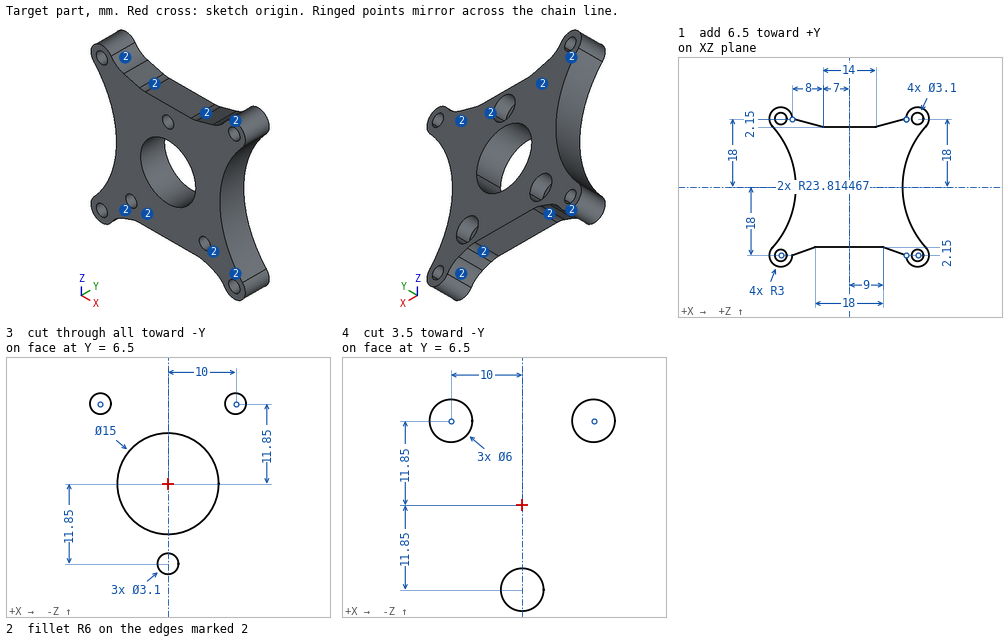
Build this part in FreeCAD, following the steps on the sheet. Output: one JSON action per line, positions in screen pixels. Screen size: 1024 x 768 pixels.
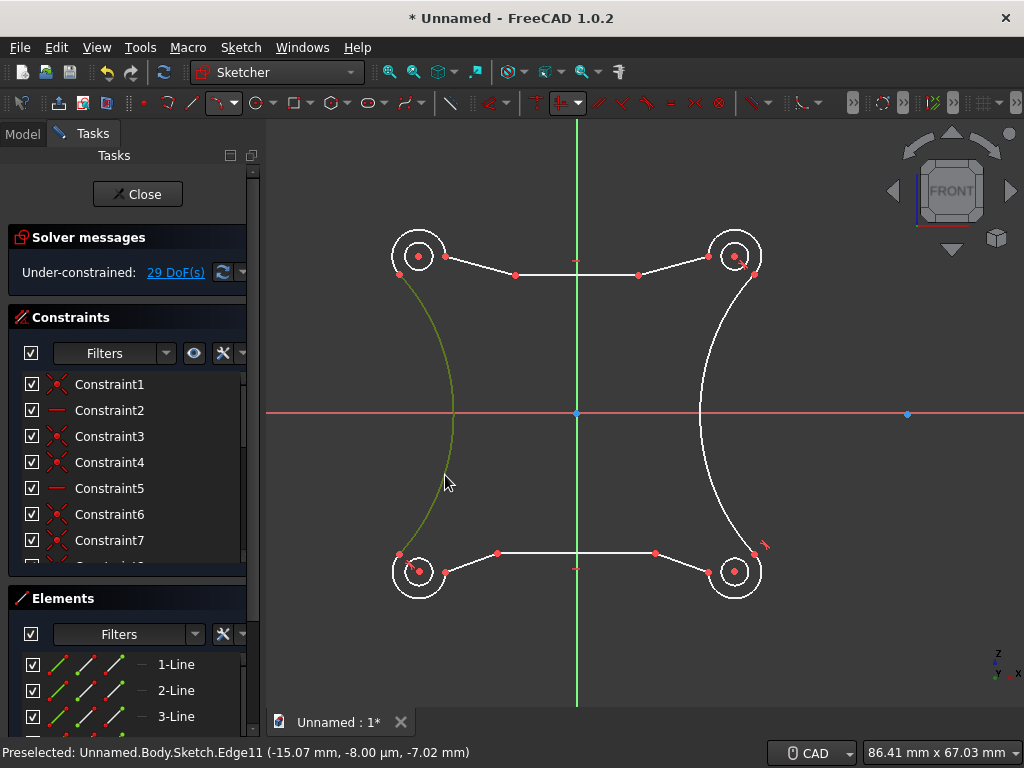
{"action": "left_click", "coordinate": [429, 232]}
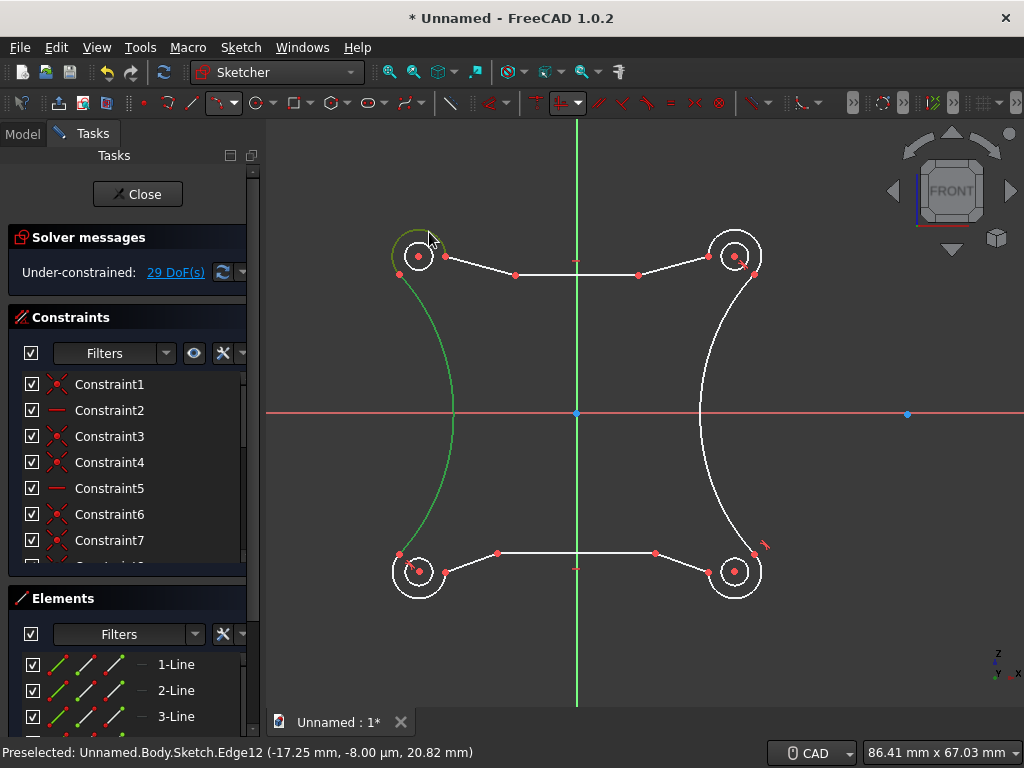
{"action": "left_click", "coordinate": [648, 104]}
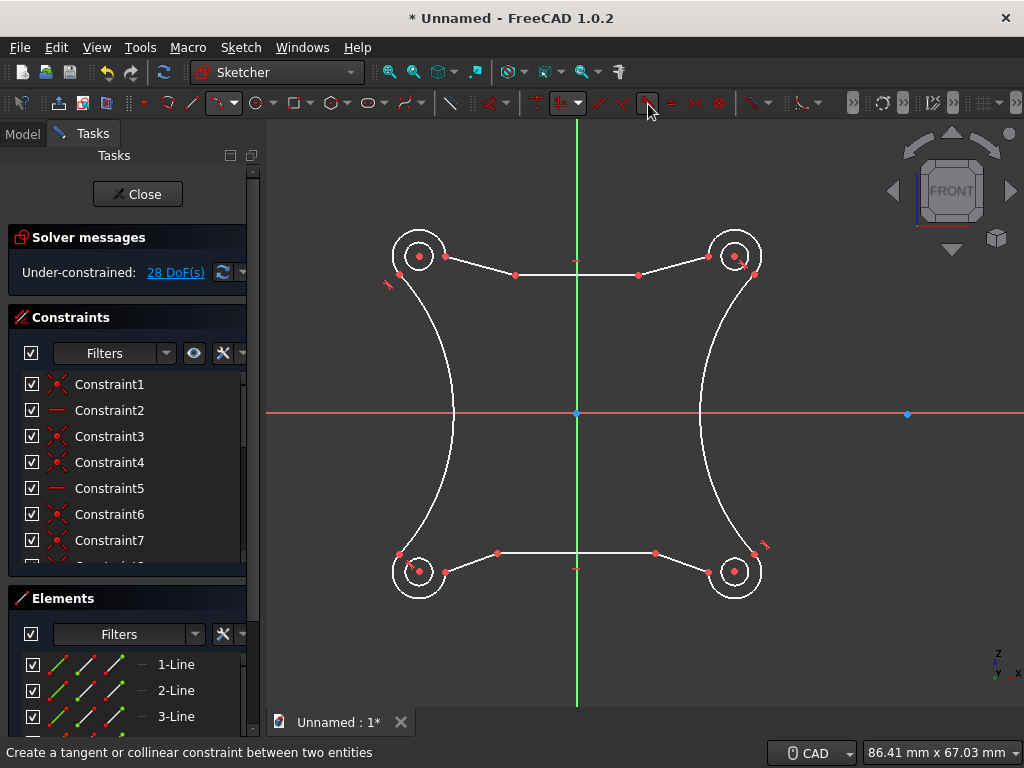
{"action": "left_click", "coordinate": [759, 245]}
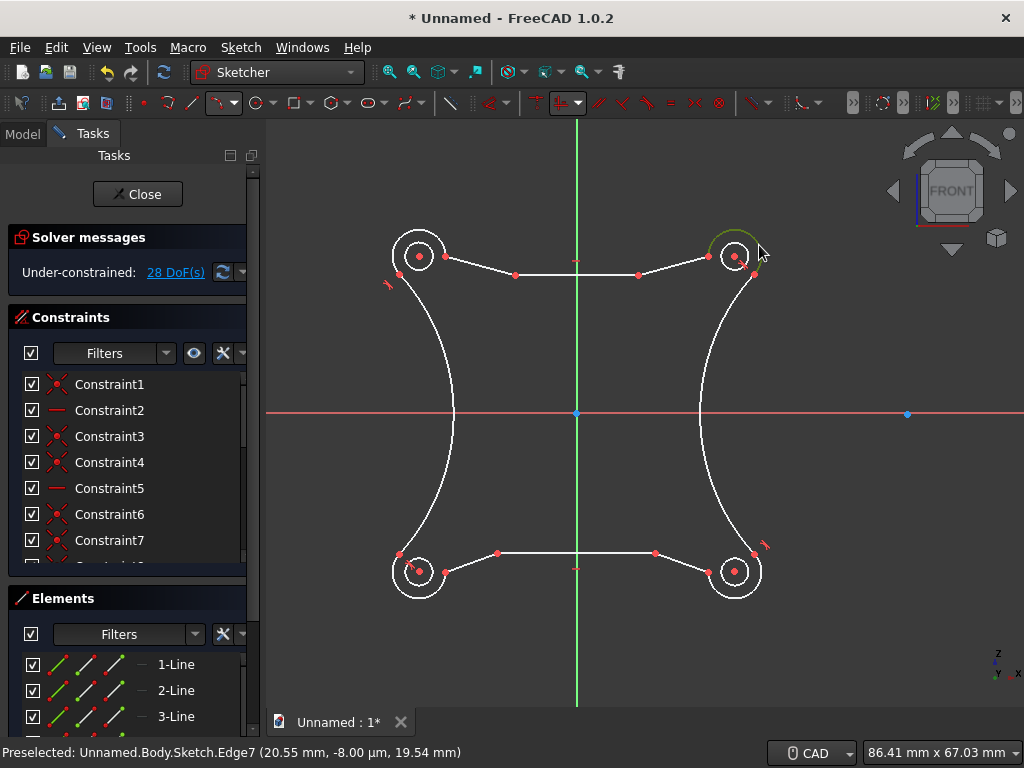
{"action": "left_click", "coordinate": [725, 596]}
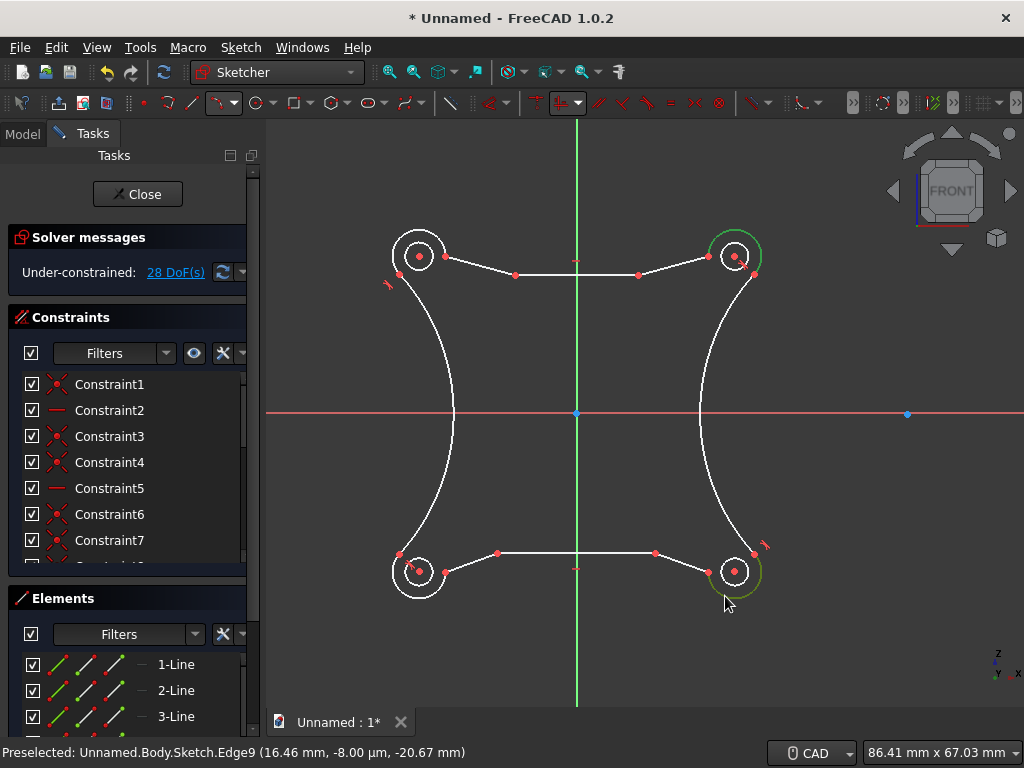
{"action": "left_click", "coordinate": [395, 583]}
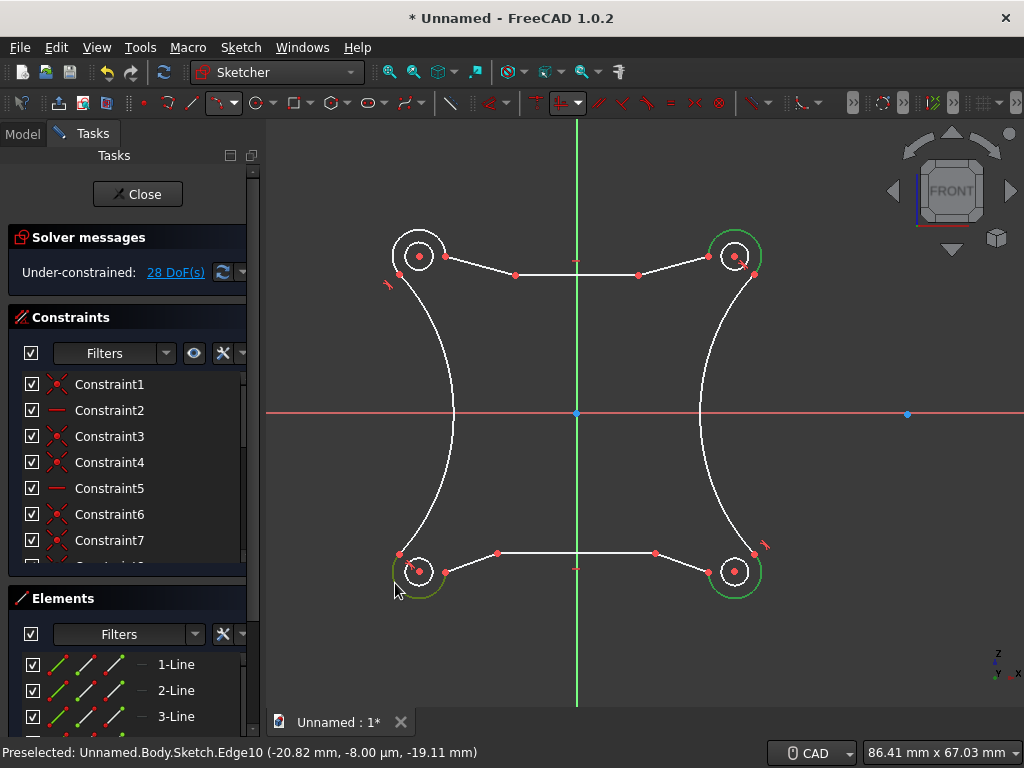
{"action": "left_click", "coordinate": [430, 232]}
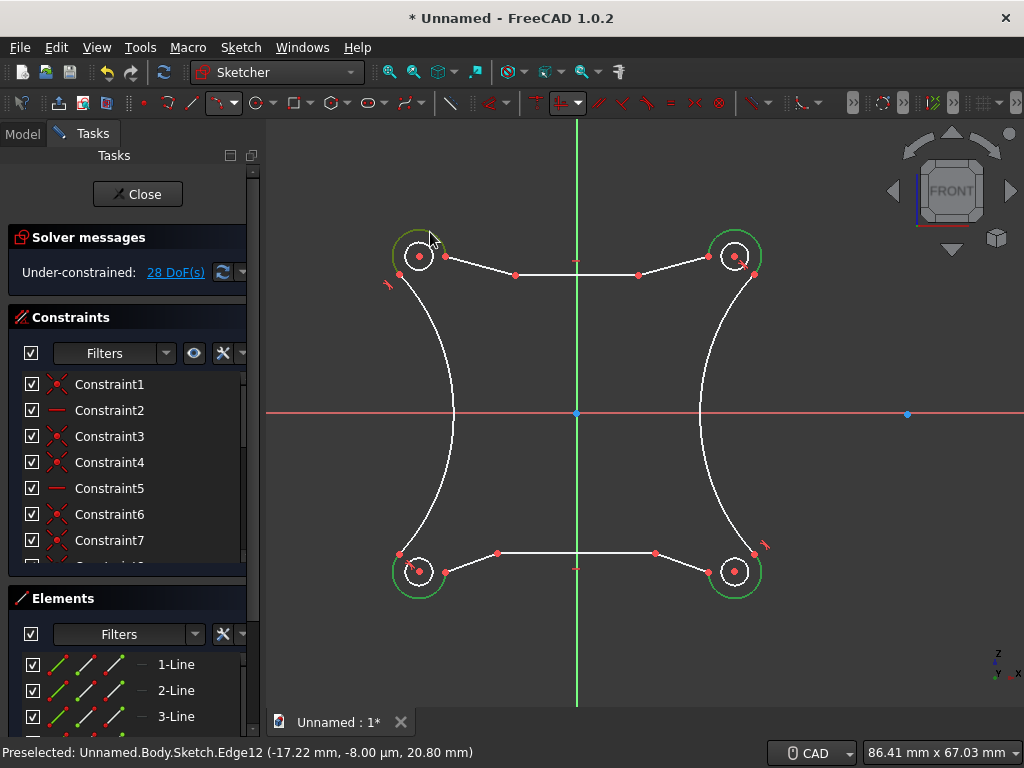
{"action": "left_click", "coordinate": [672, 104]}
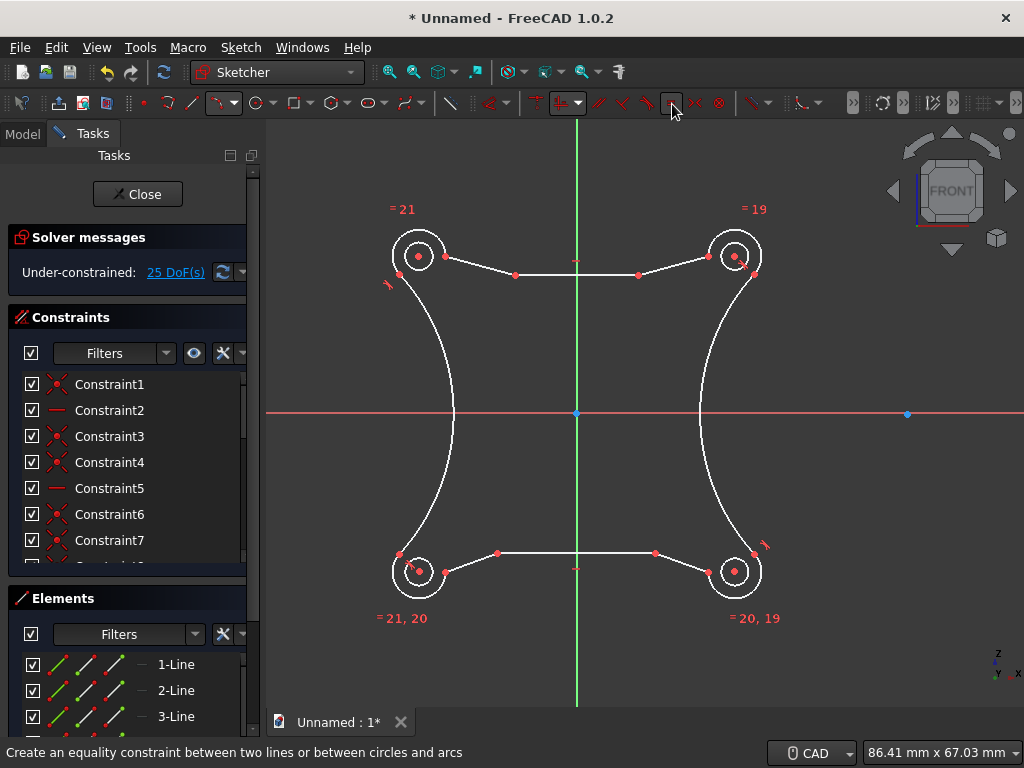
{"action": "left_click", "coordinate": [709, 354]}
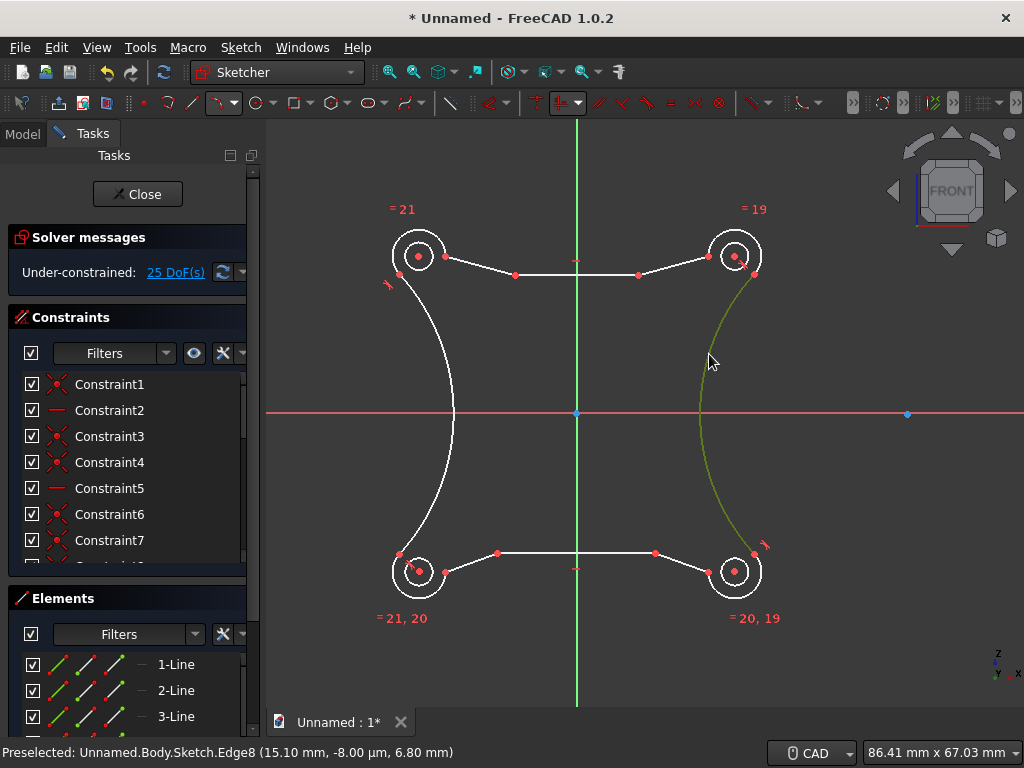
{"action": "left_click", "coordinate": [445, 475]}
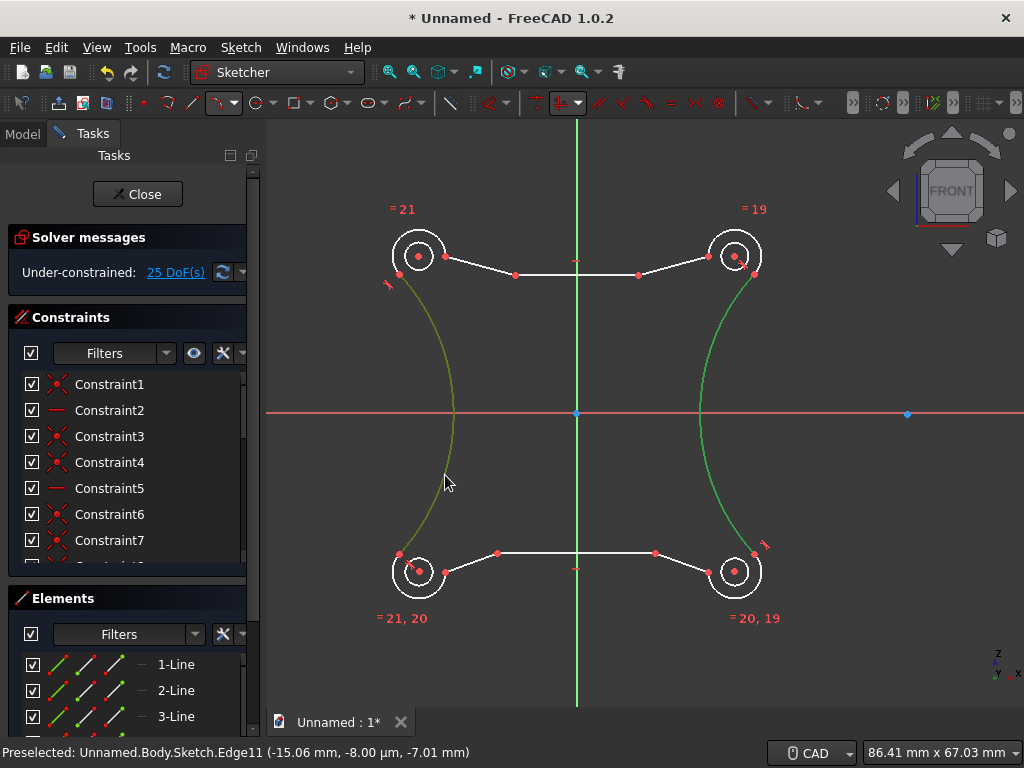
{"action": "left_click", "coordinate": [672, 104]}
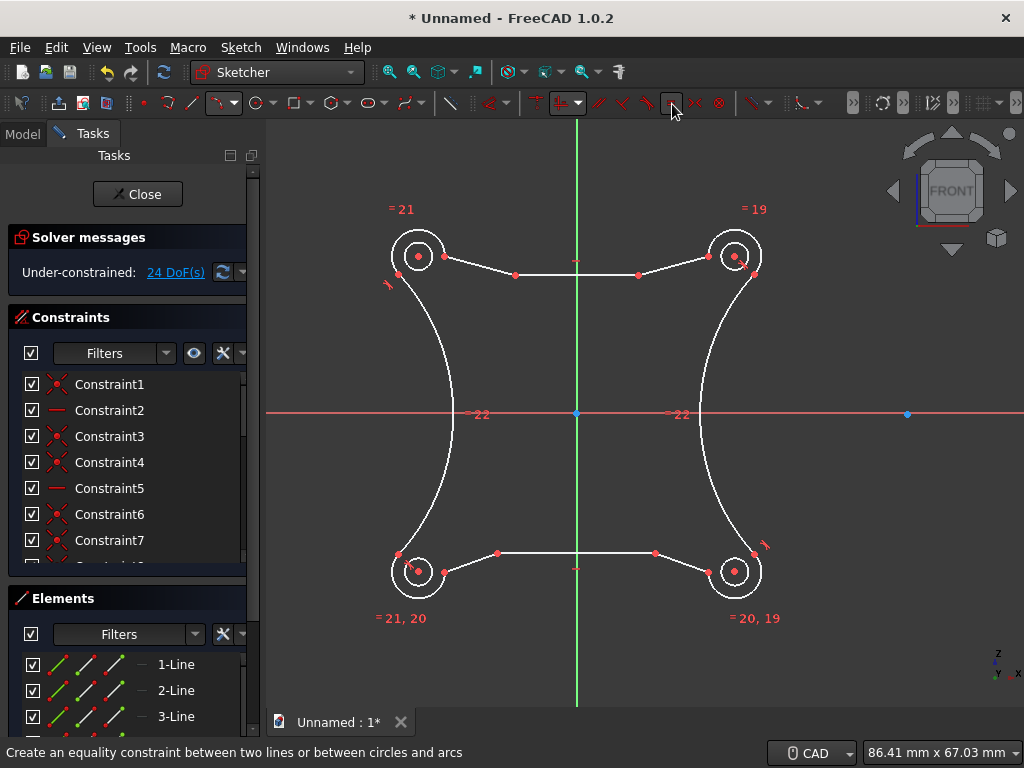
{"action": "left_click", "coordinate": [744, 247]}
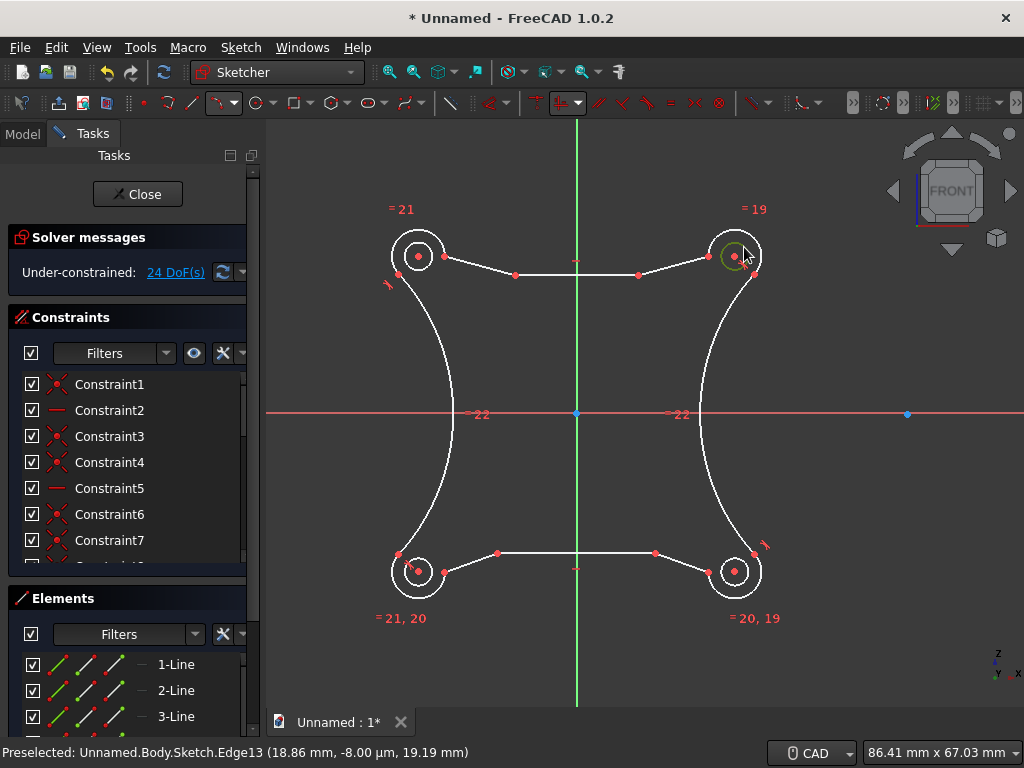
{"action": "left_click", "coordinate": [428, 247]}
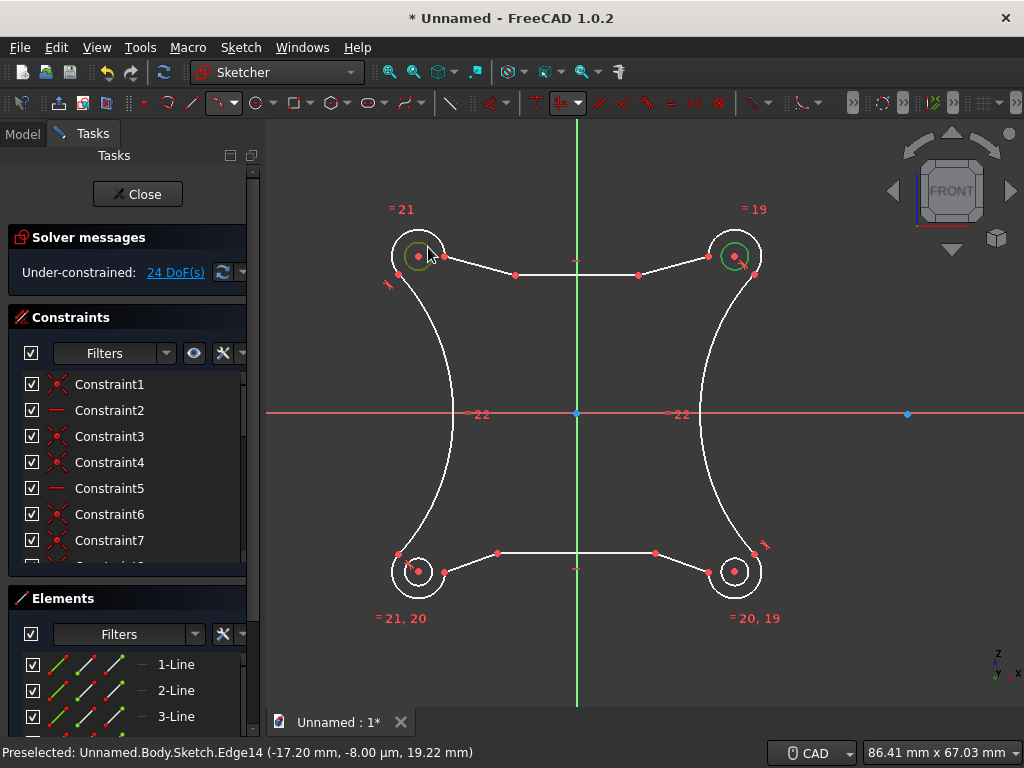
{"action": "left_click", "coordinate": [744, 562]}